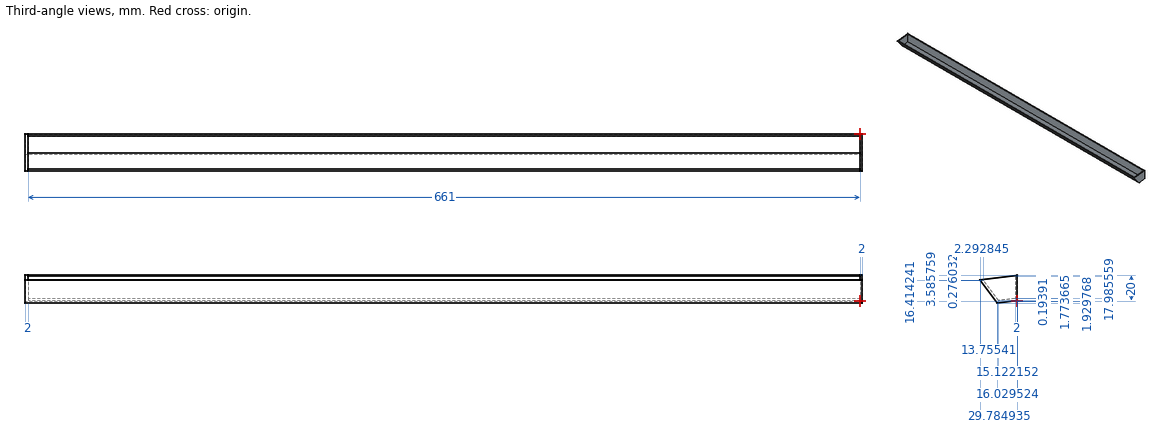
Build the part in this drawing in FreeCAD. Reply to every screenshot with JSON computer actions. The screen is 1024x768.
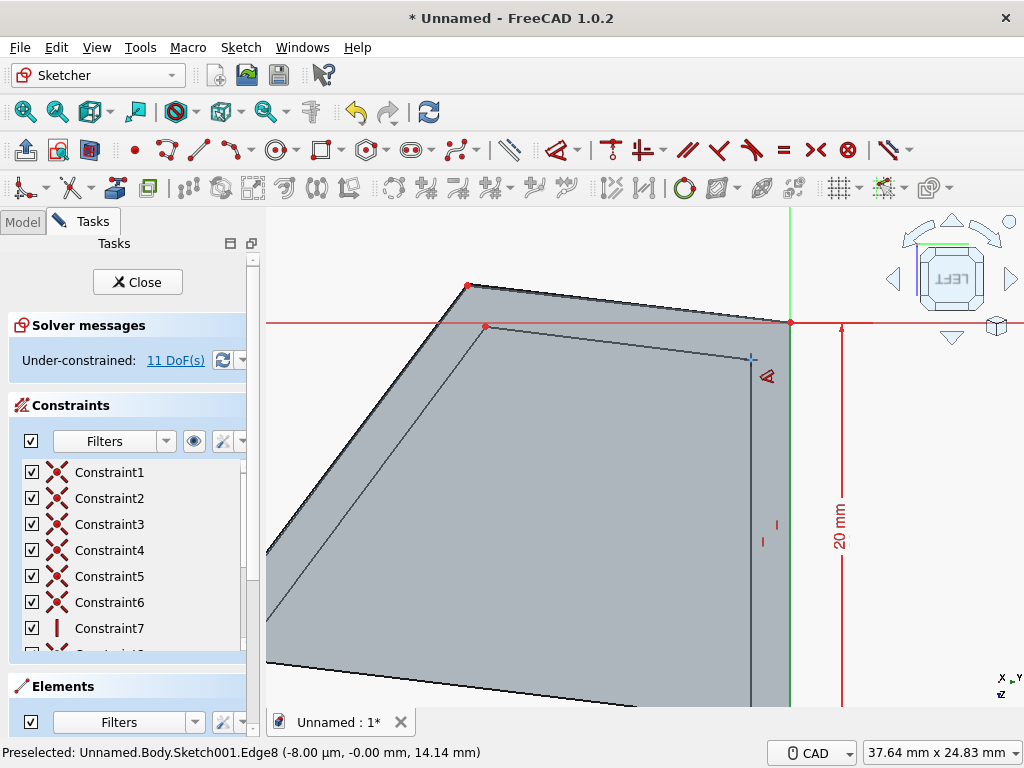
{"action": "left_click", "coordinate": [751, 360]}
{"action": "left_click", "coordinate": [771, 289]}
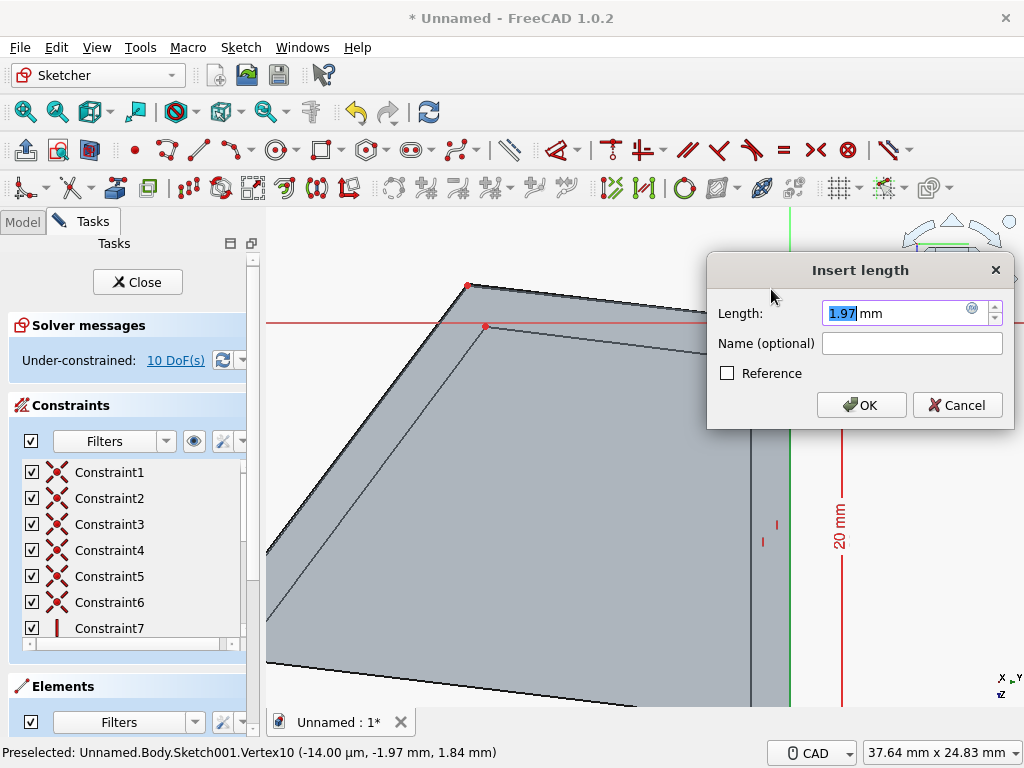
{"action": "type", "text": "2"}
{"action": "key", "text": "Return"}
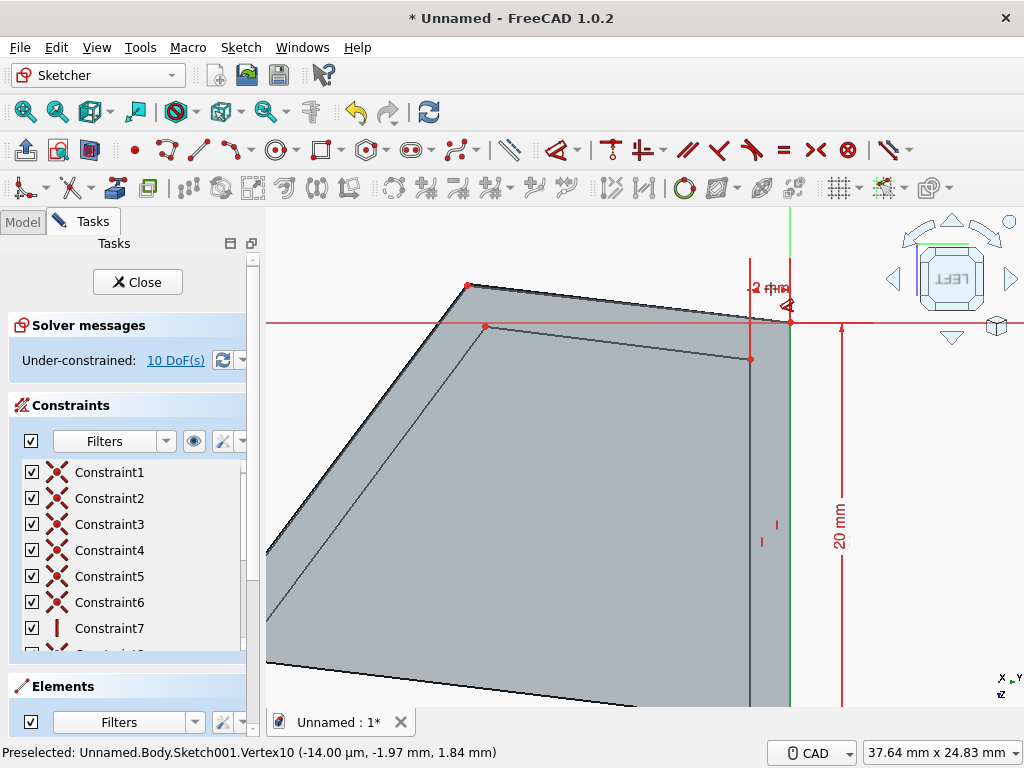
{"action": "scroll", "coordinate": [486, 327], "scroll_direction": "up", "scroll_amount": 12}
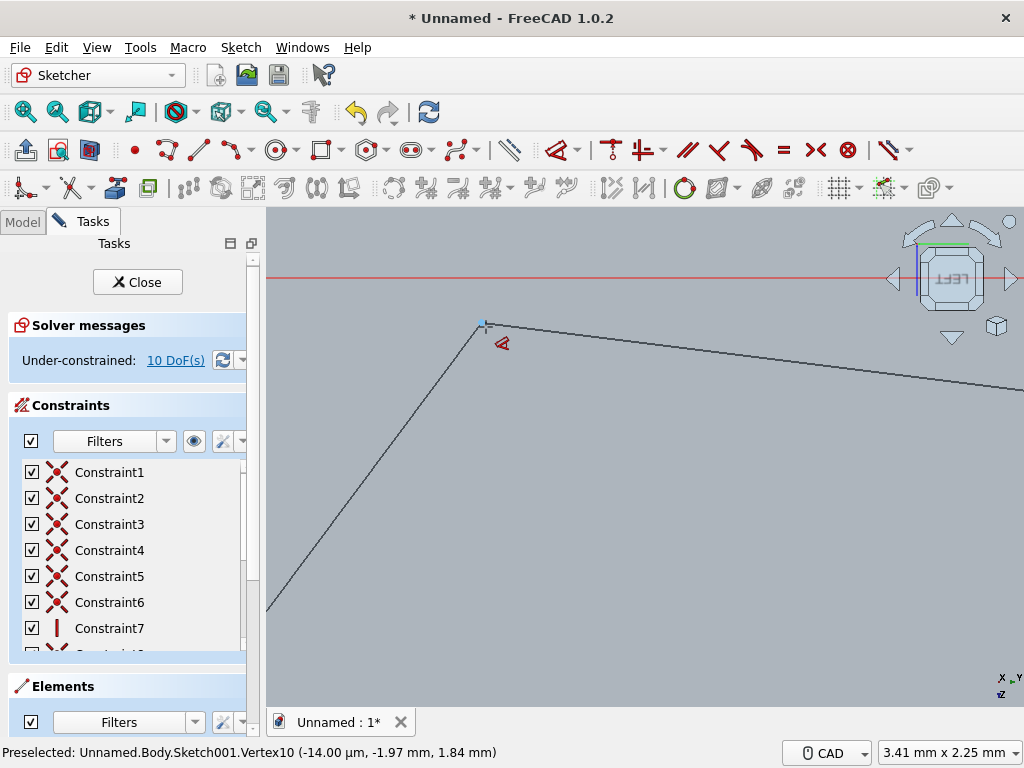
{"action": "left_click", "coordinate": [482, 323]}
{"action": "left_click", "coordinate": [448, 300]}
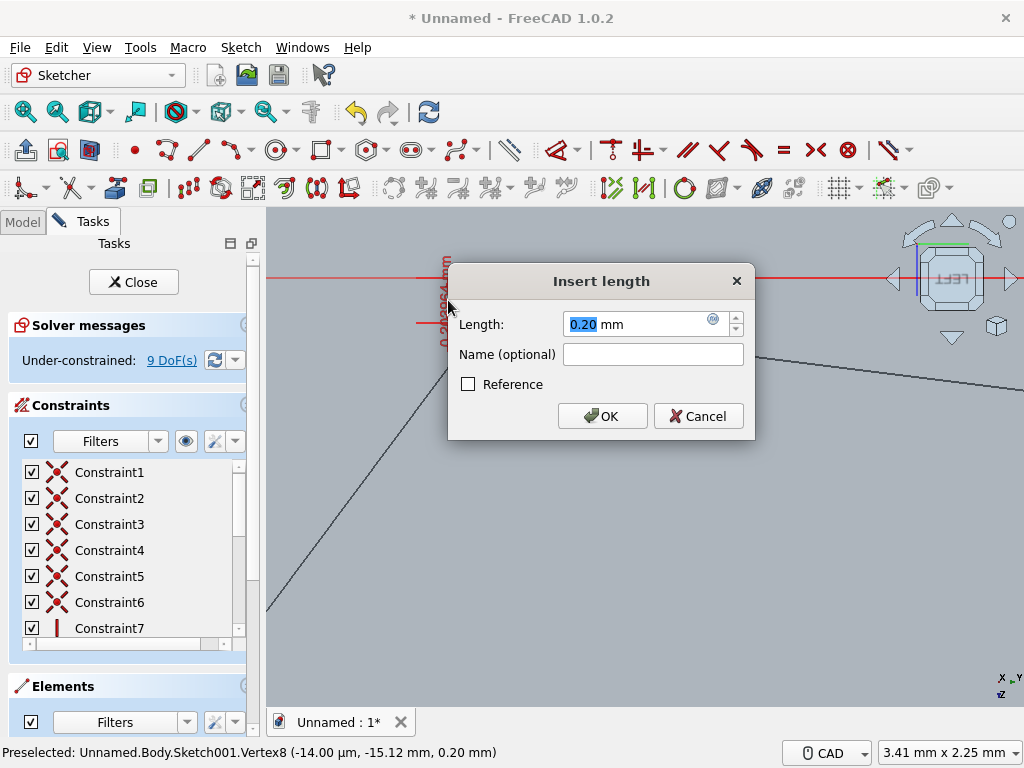
{"action": "type", "text": "0.19391"}
{"action": "key", "text": "Return"}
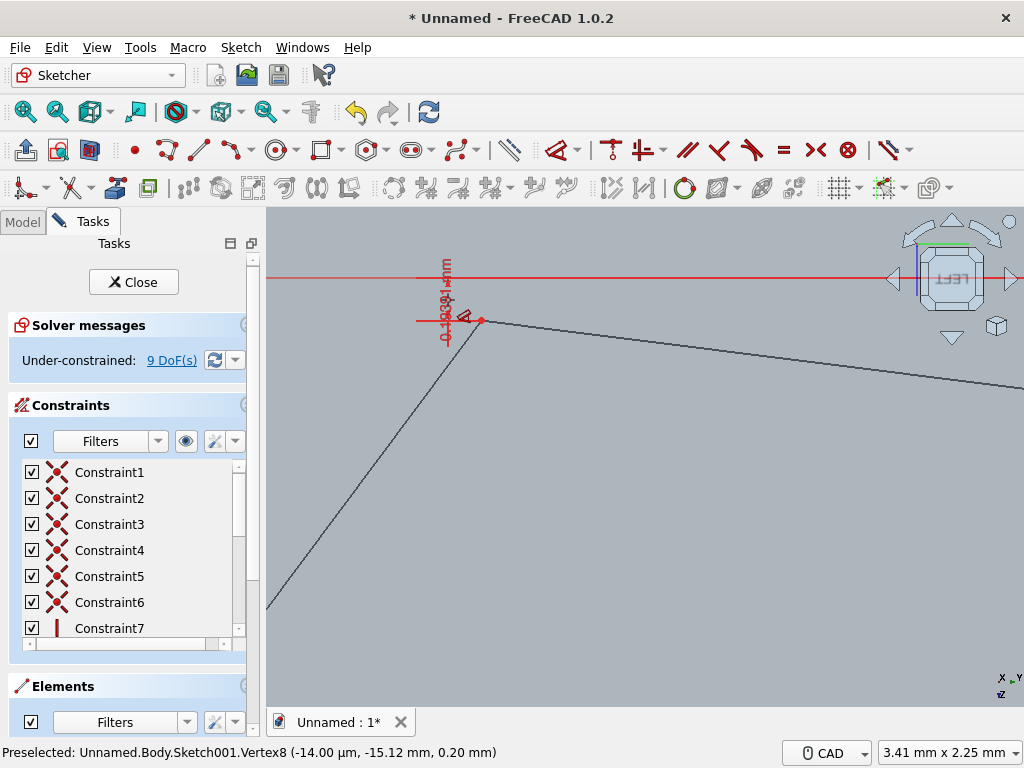
{"action": "scroll", "coordinate": [579, 339], "scroll_direction": "down", "scroll_amount": 14}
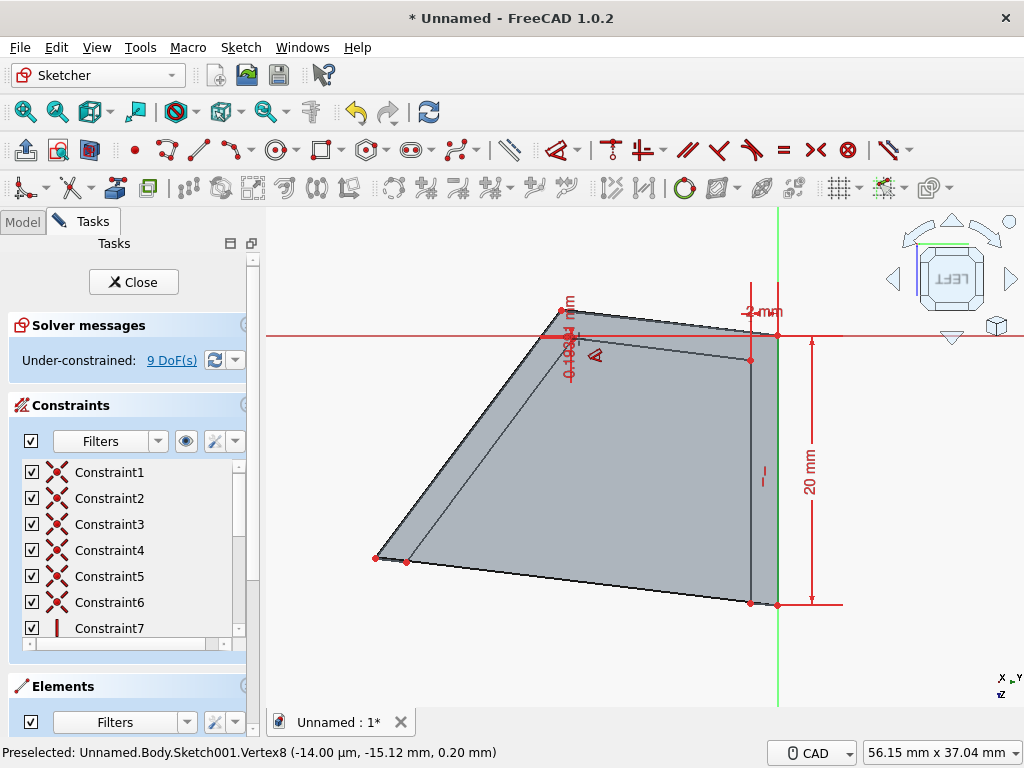
{"action": "left_click", "coordinate": [751, 433]}
{"action": "left_click", "coordinate": [717, 482]}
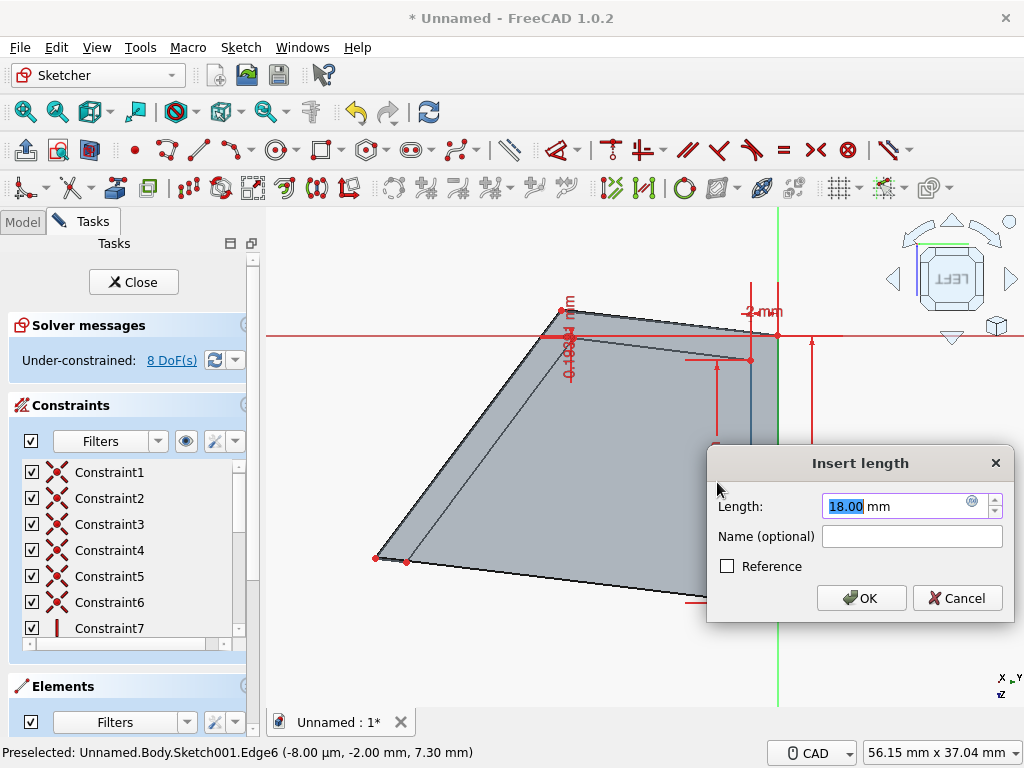
{"action": "type", "text": "17.985559"}
{"action": "key", "text": "Return"}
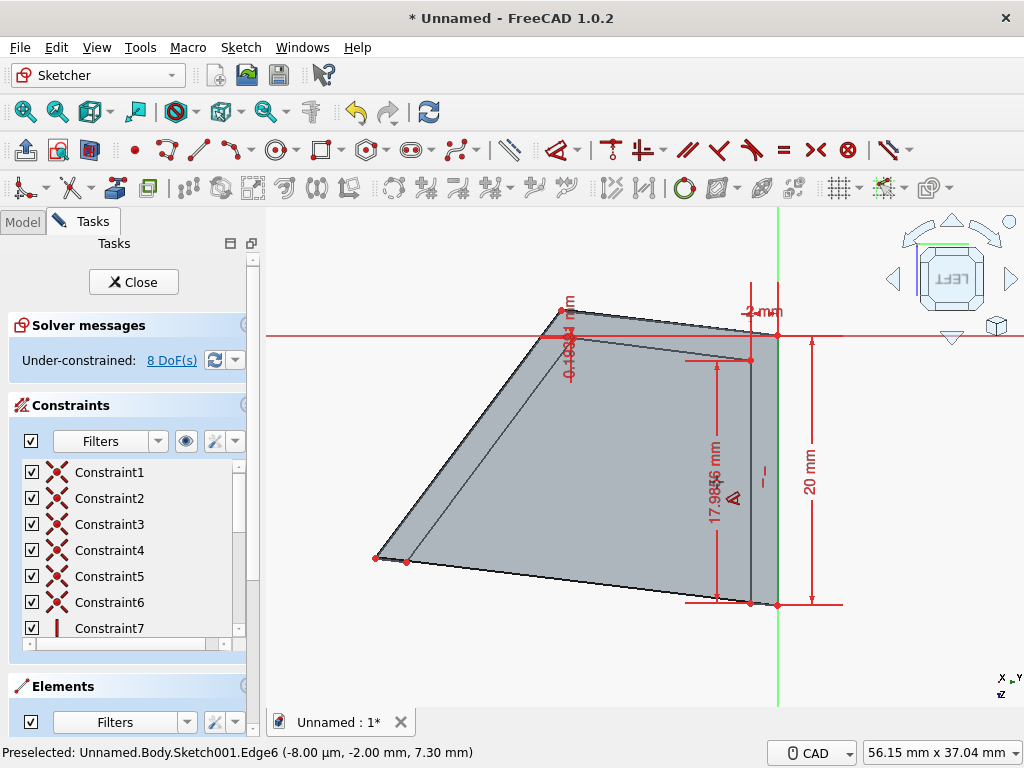
{"action": "scroll", "coordinate": [561, 311], "scroll_direction": "up", "scroll_amount": 3}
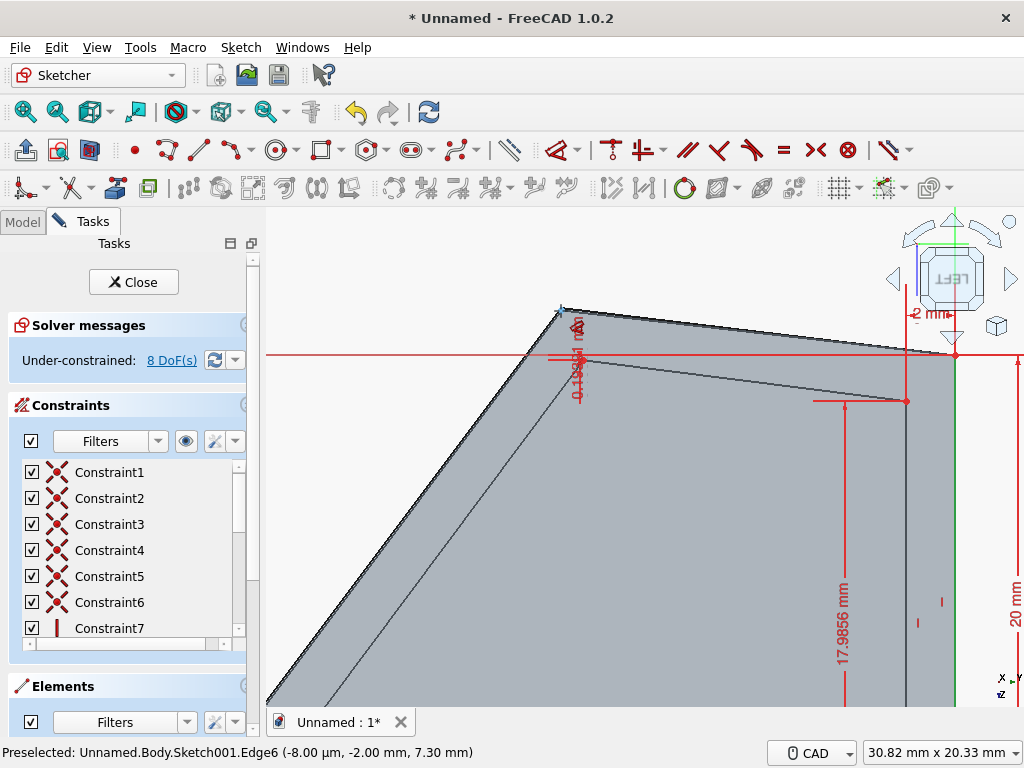
{"action": "left_click", "coordinate": [562, 310]}
{"action": "left_click", "coordinate": [528, 333]}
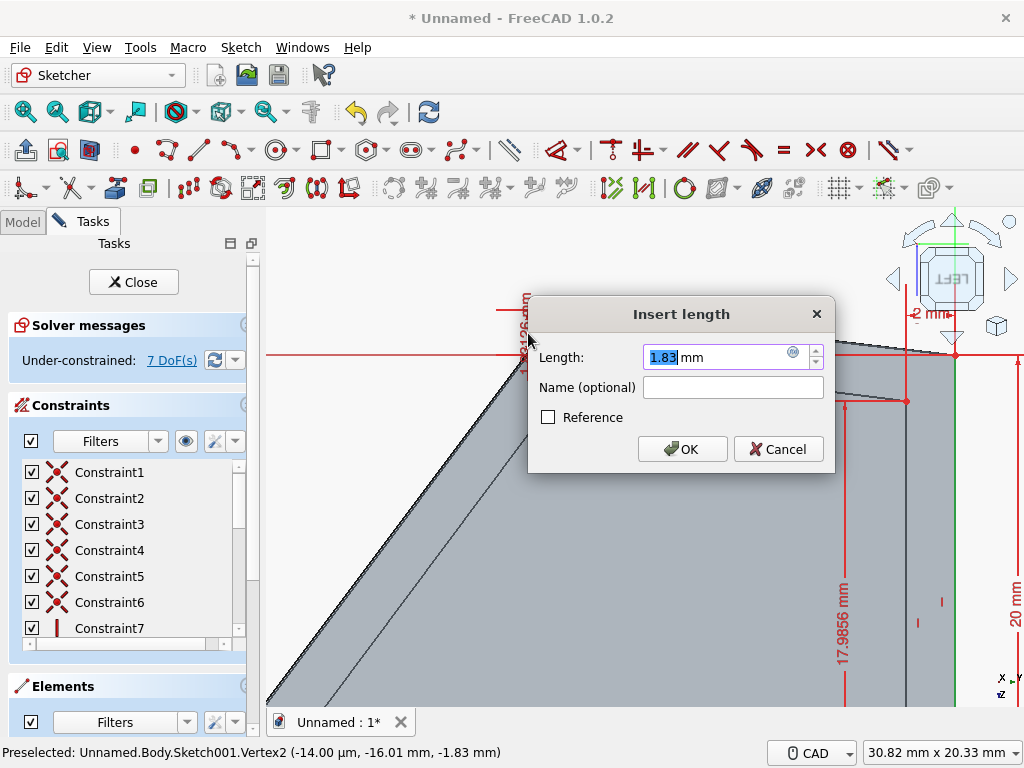
{"action": "type", "text": "1.929768"}
{"action": "key", "text": "Return"}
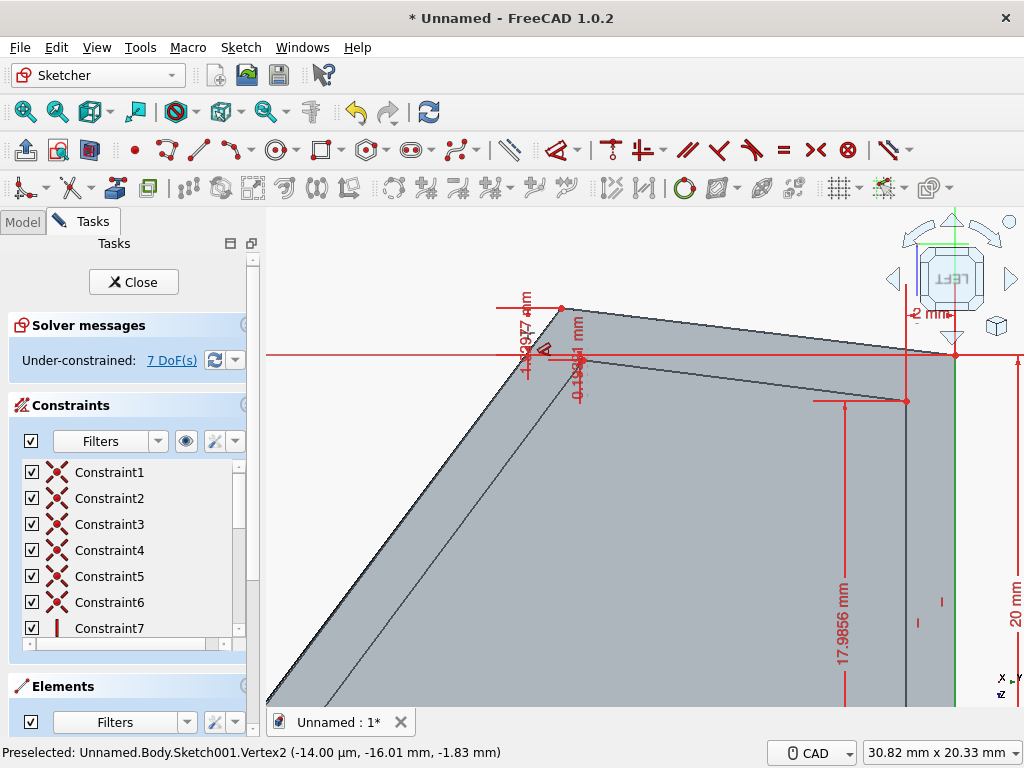
{"action": "scroll", "coordinate": [561, 310], "scroll_direction": "down", "scroll_amount": 3}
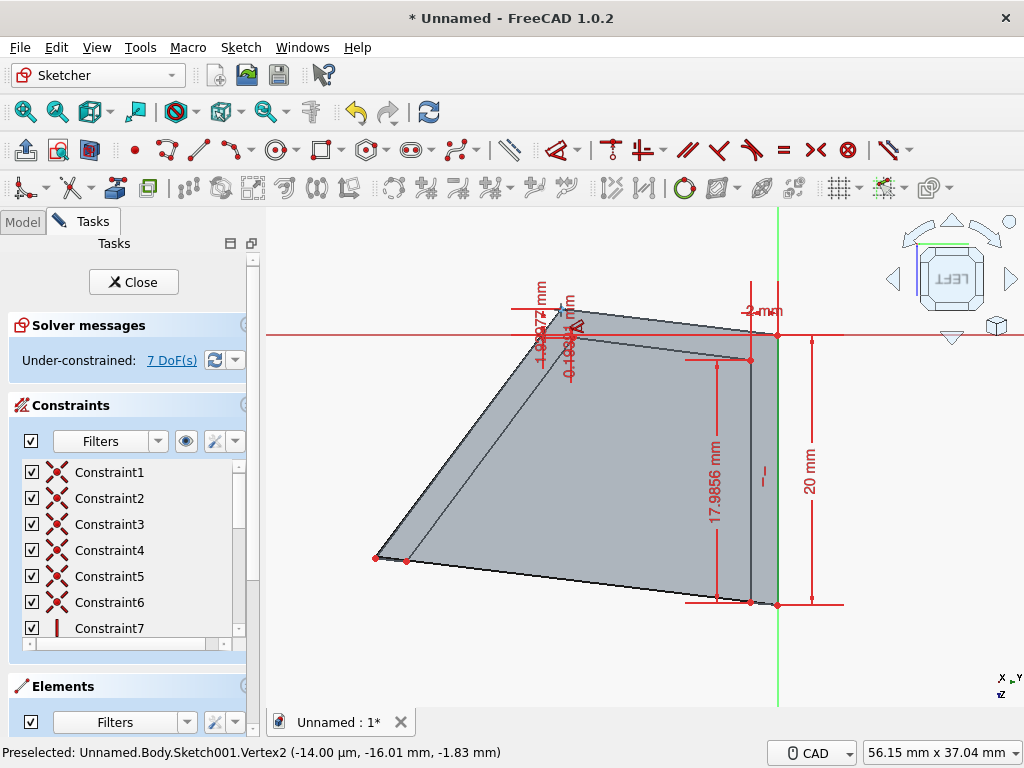
{"action": "scroll", "coordinate": [751, 360], "scroll_direction": "up", "scroll_amount": 3}